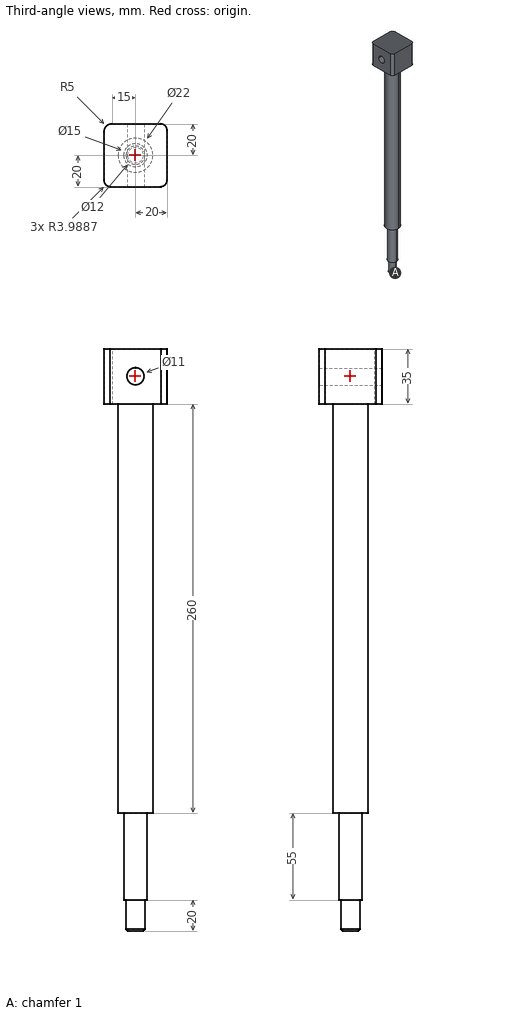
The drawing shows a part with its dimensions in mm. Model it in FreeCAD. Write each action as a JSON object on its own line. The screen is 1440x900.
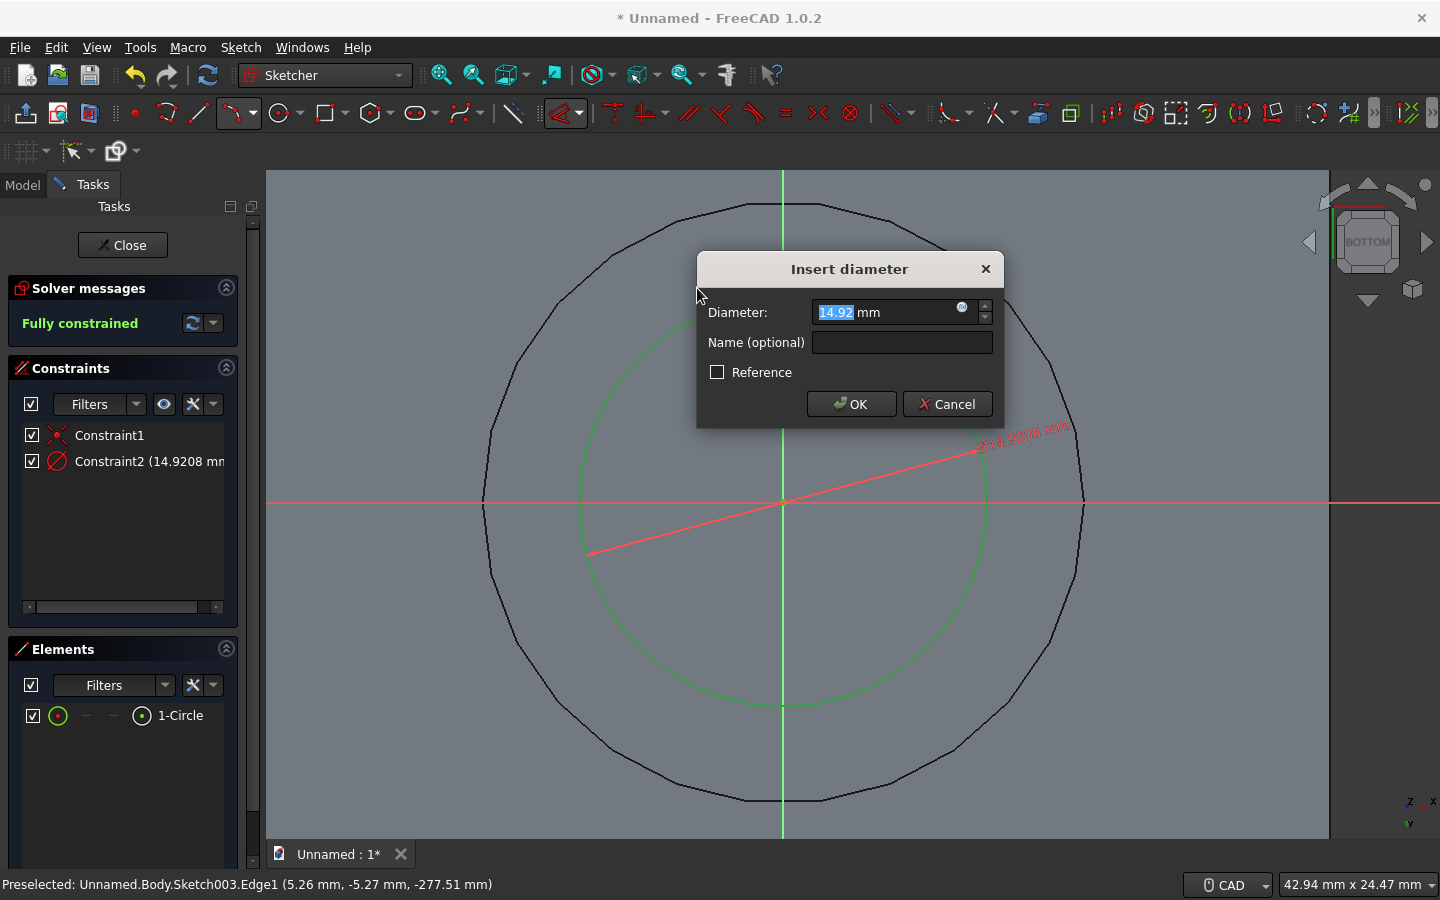
{"action": "type", "text": "15"}
{"action": "key", "text": "Return"}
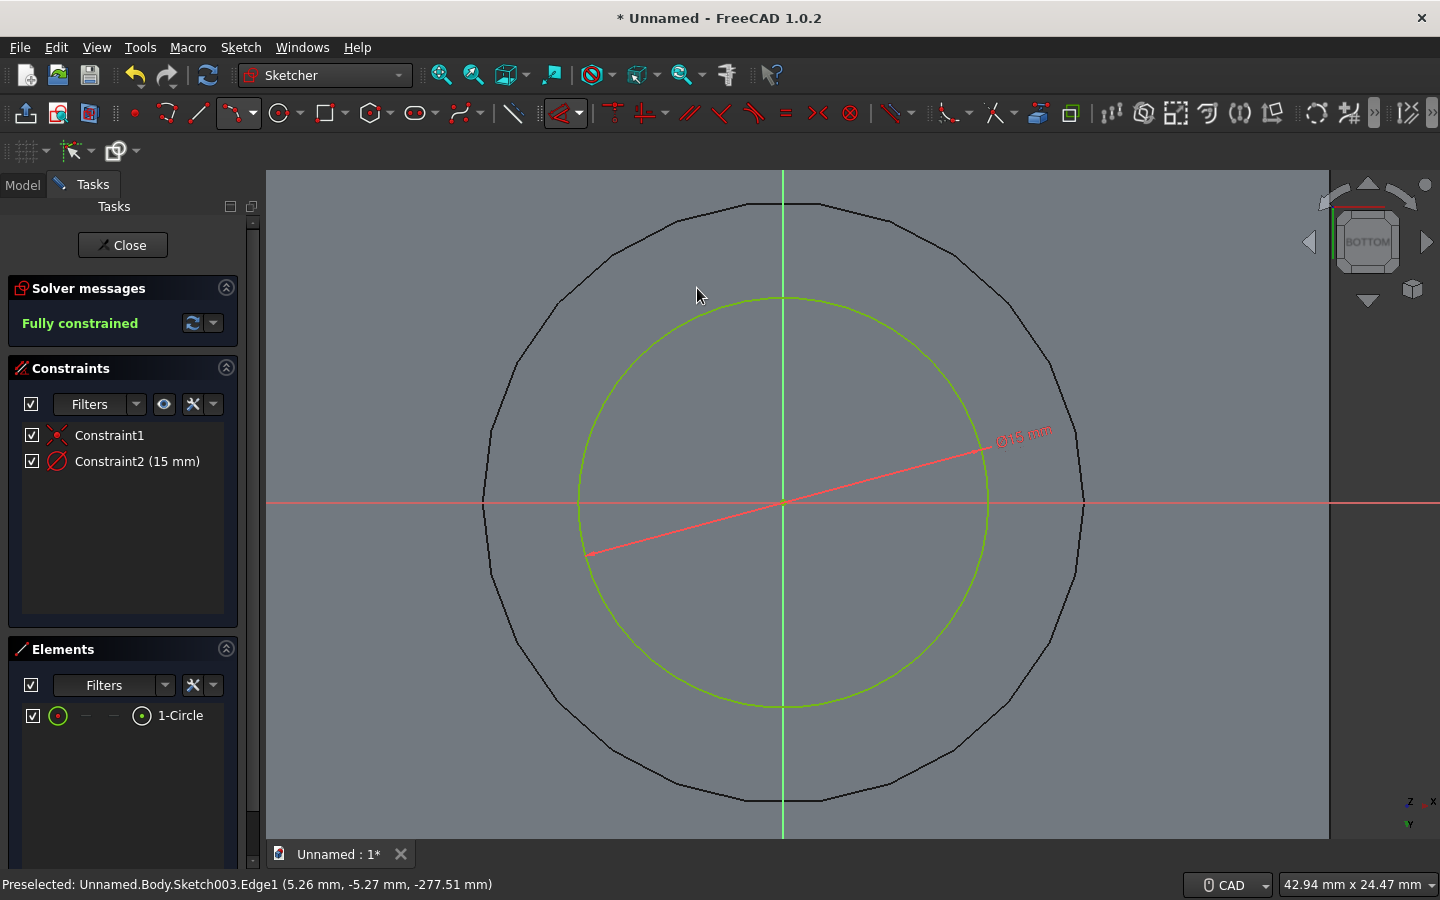
{"action": "left_click", "coordinate": [123, 245]}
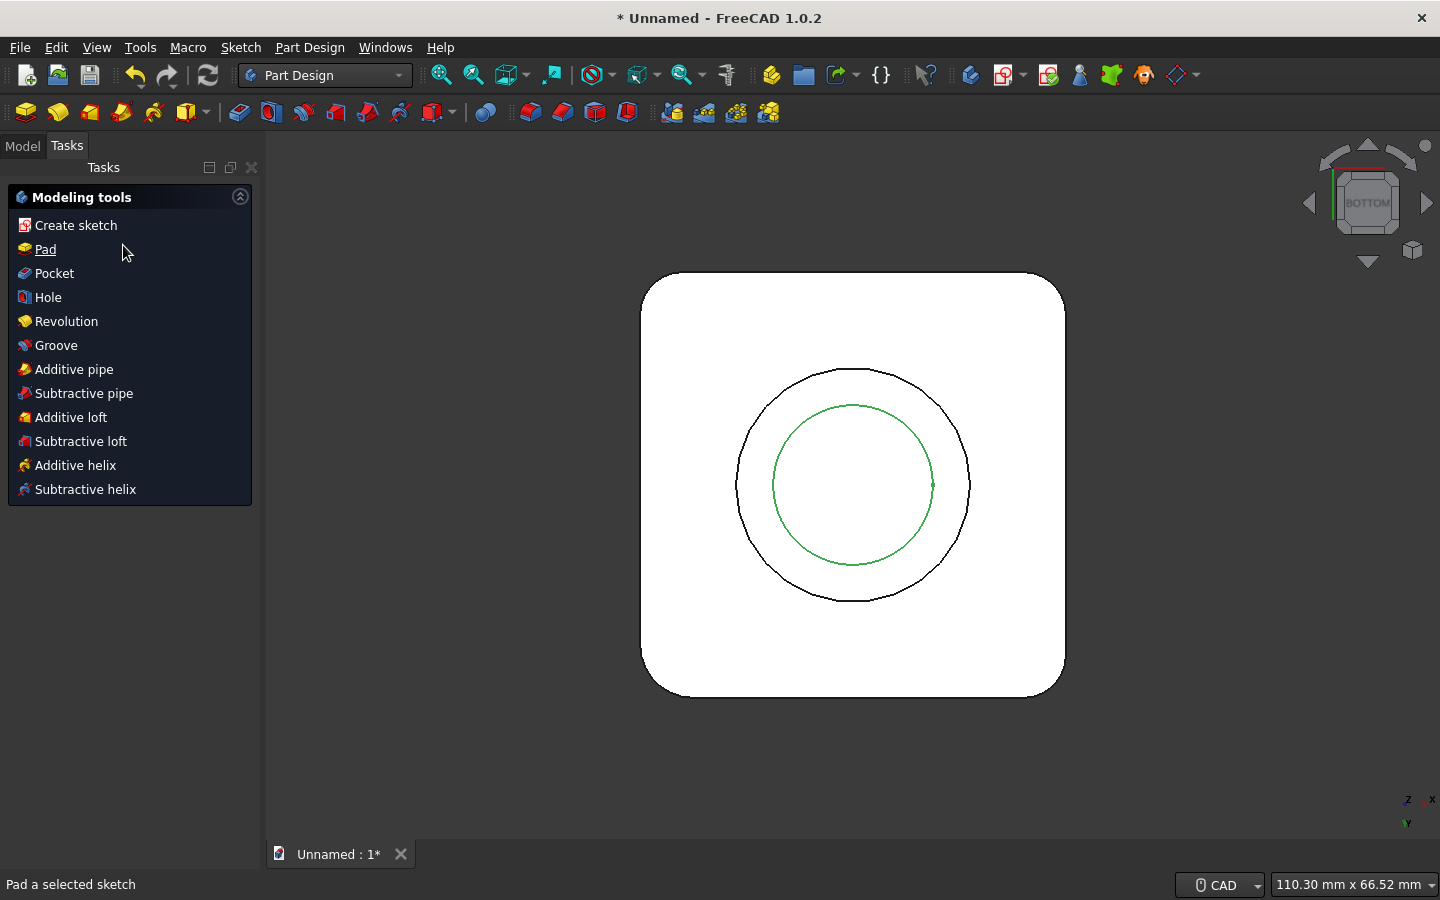
{"action": "left_click", "coordinate": [26, 112]}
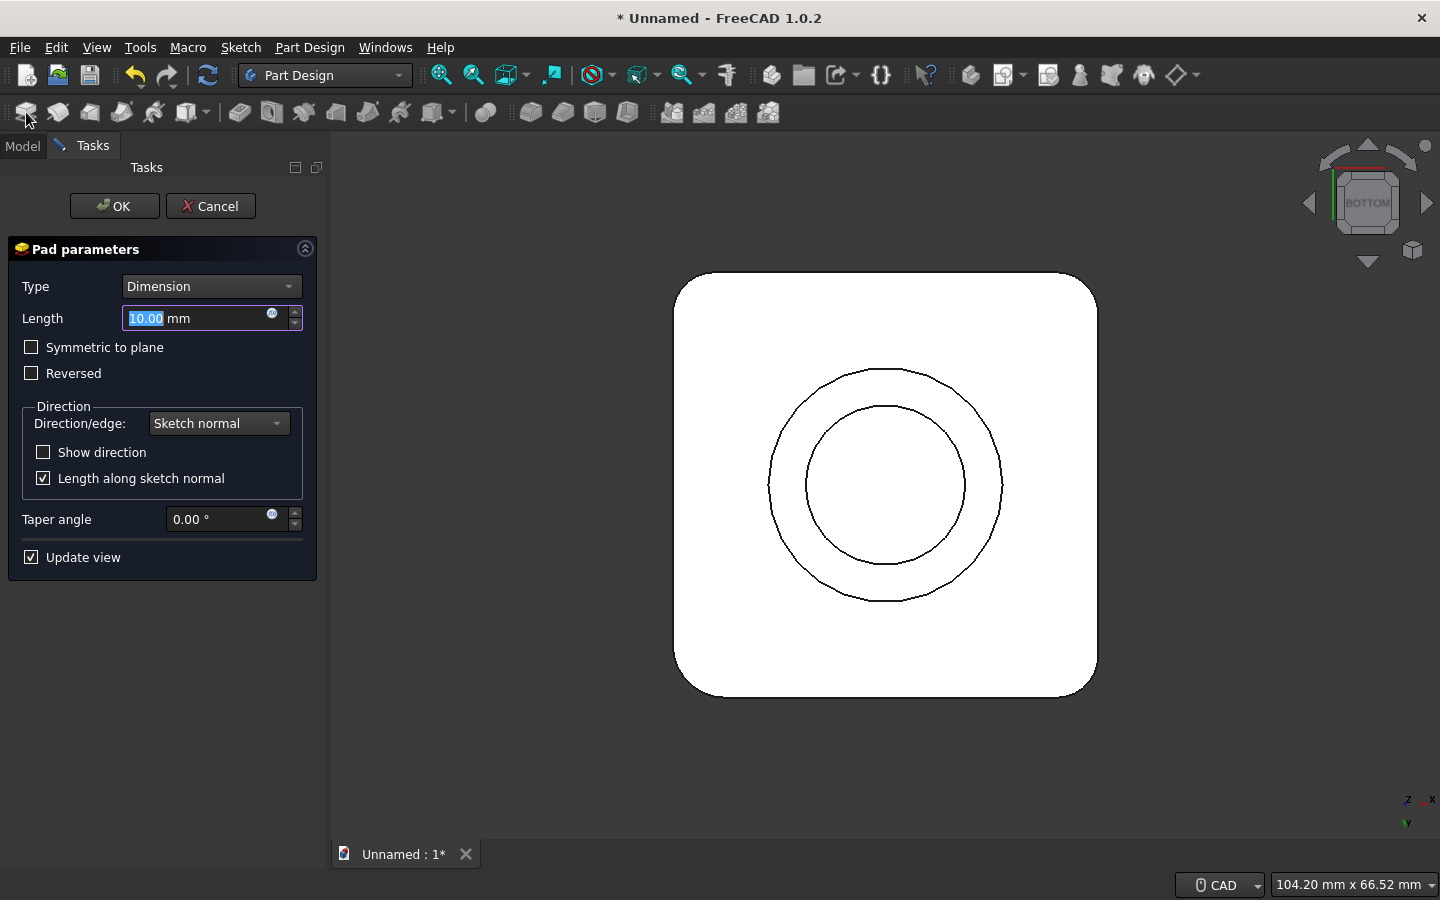
{"action": "type", "text": "55"}
{"action": "key", "text": "Tab"}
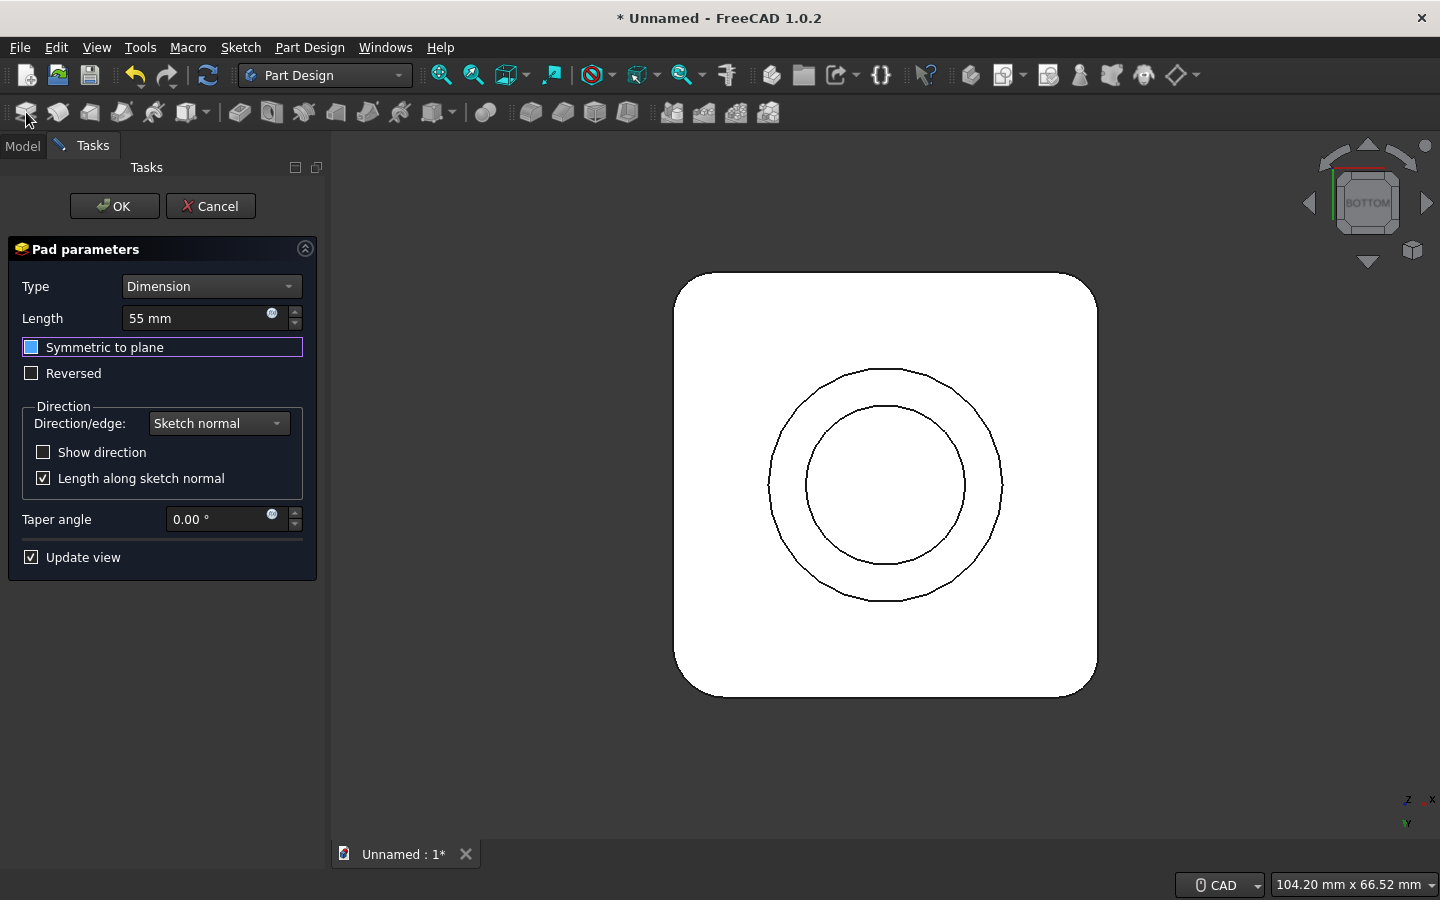
{"action": "left_click", "coordinate": [115, 206]}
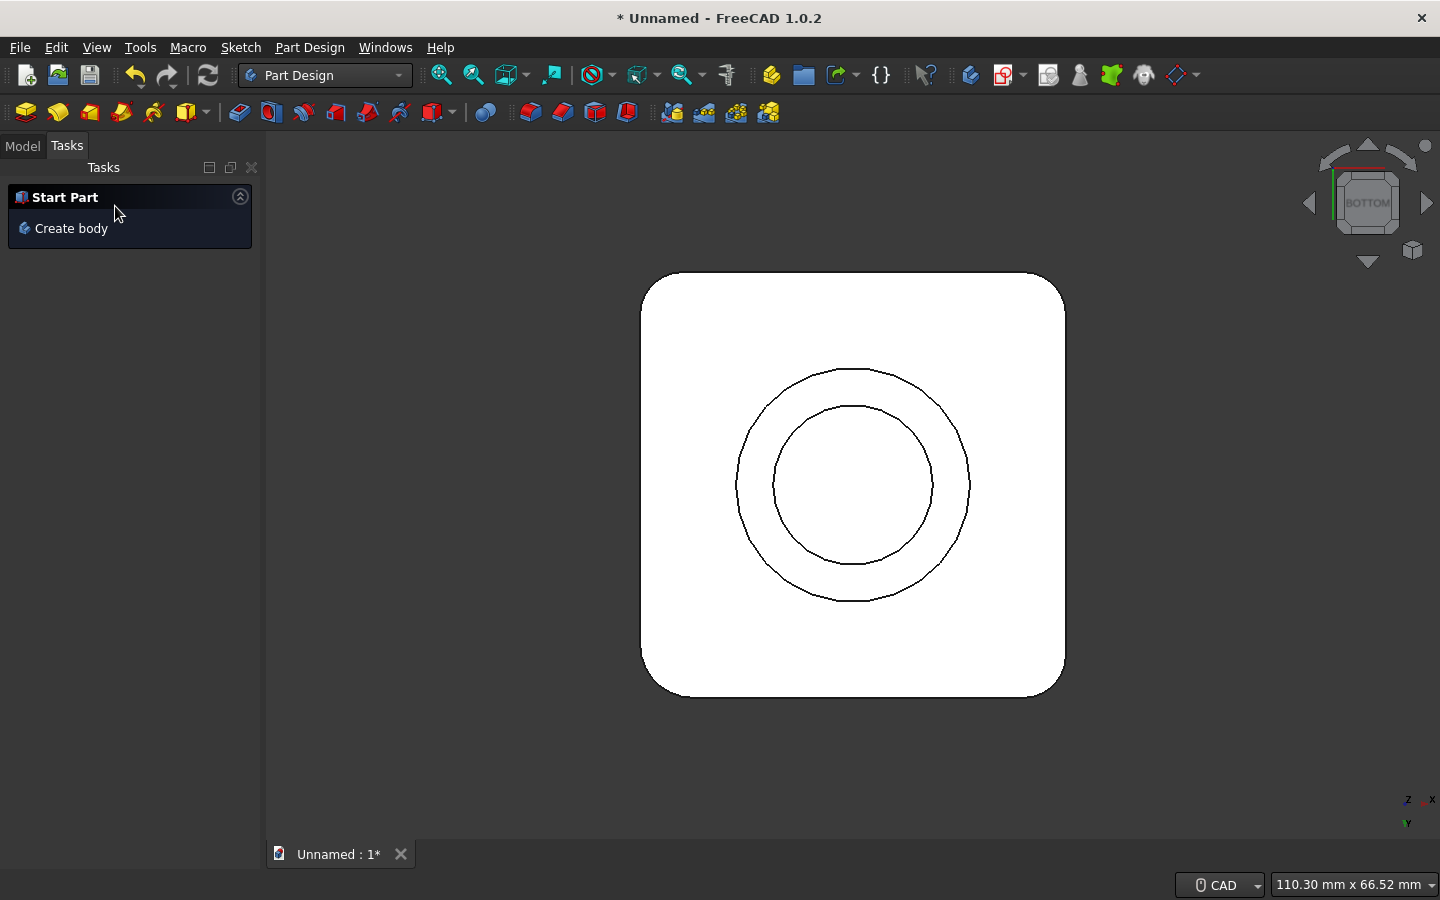
{"action": "left_click", "coordinate": [853, 484]}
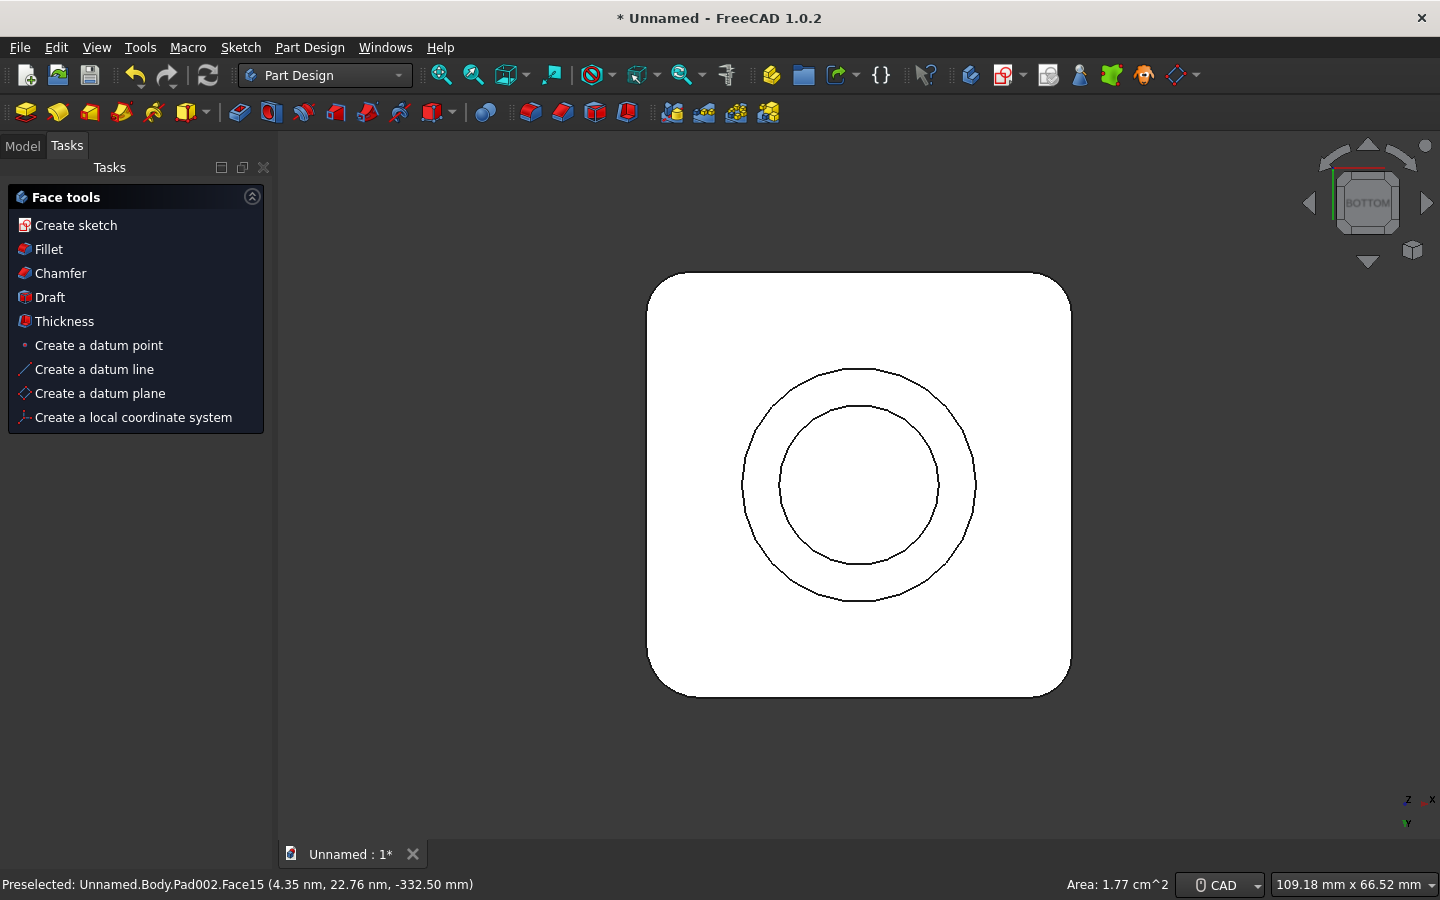
{"action": "left_click", "coordinate": [1004, 76]}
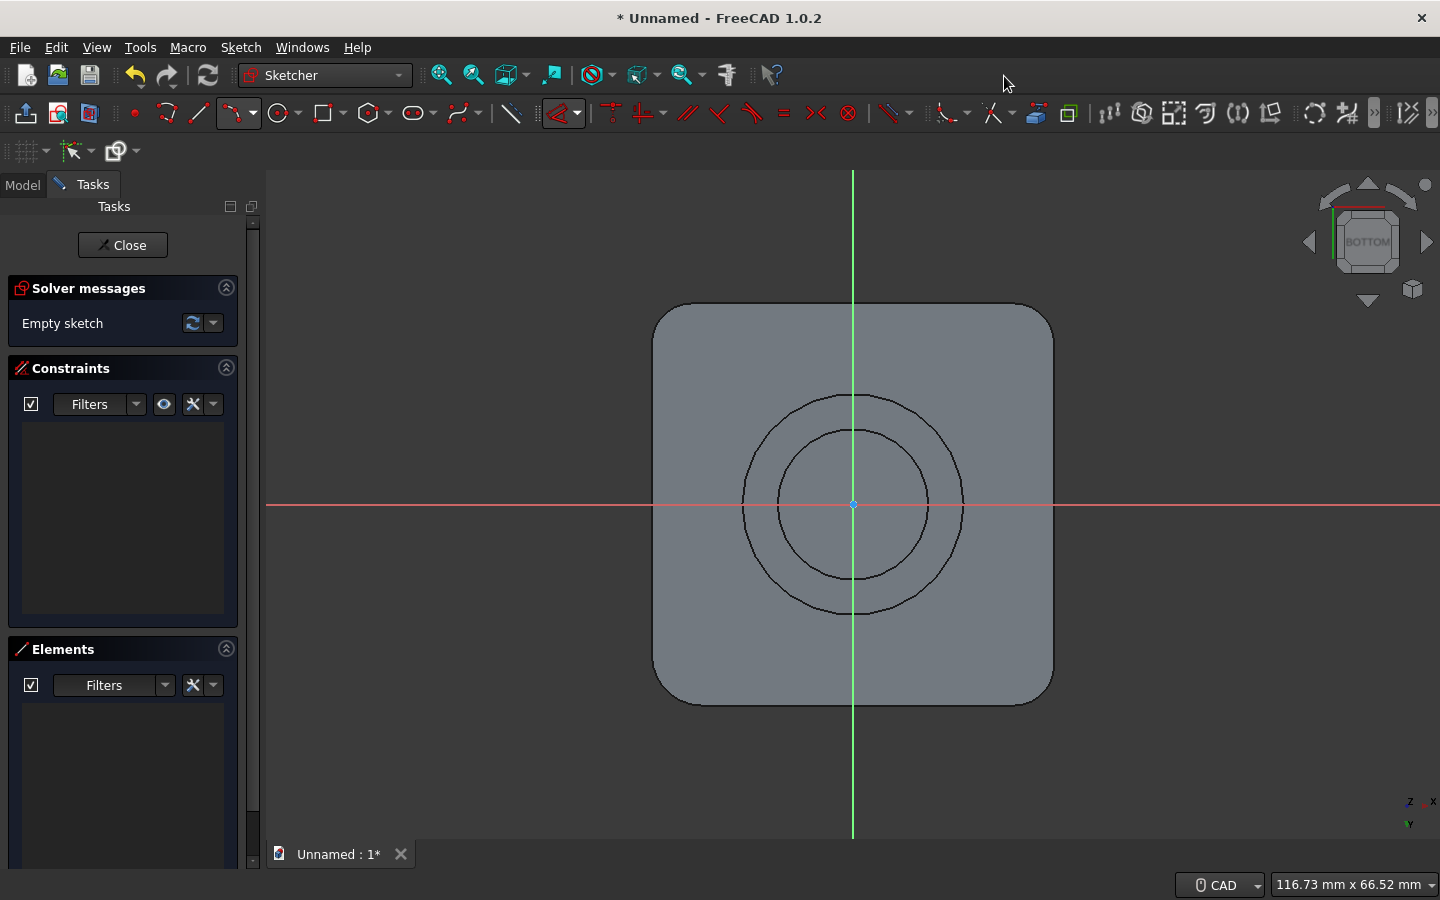
{"action": "scroll", "coordinate": [883, 505], "scroll_direction": "up", "scroll_amount": 6}